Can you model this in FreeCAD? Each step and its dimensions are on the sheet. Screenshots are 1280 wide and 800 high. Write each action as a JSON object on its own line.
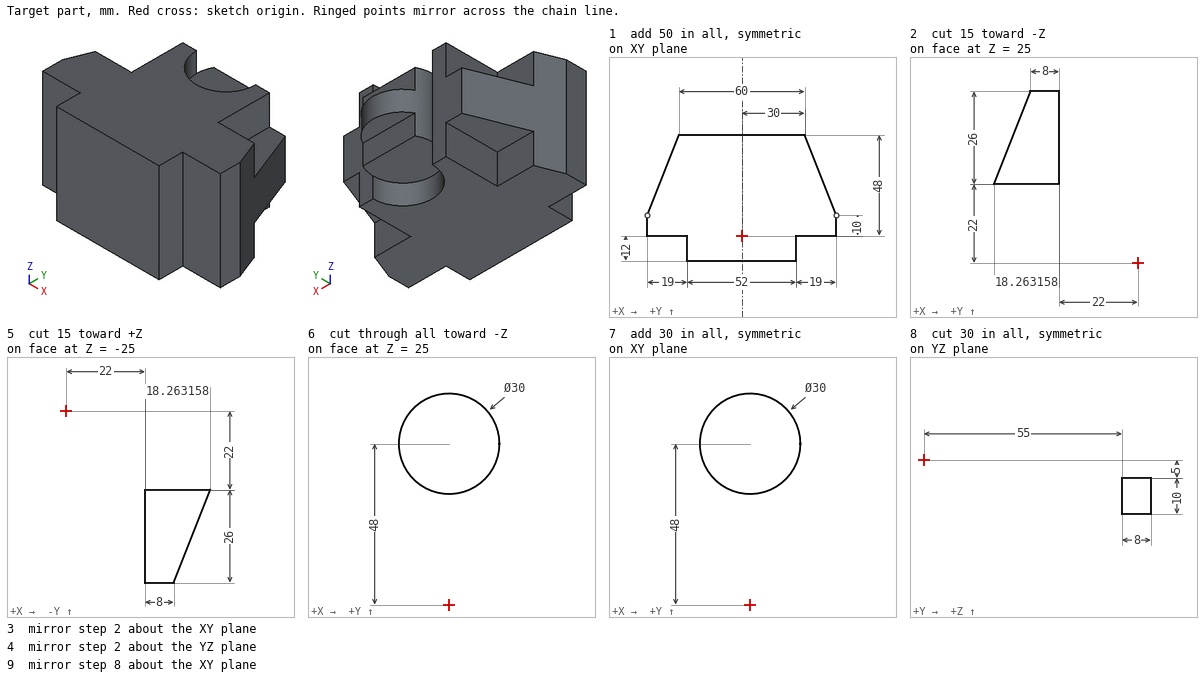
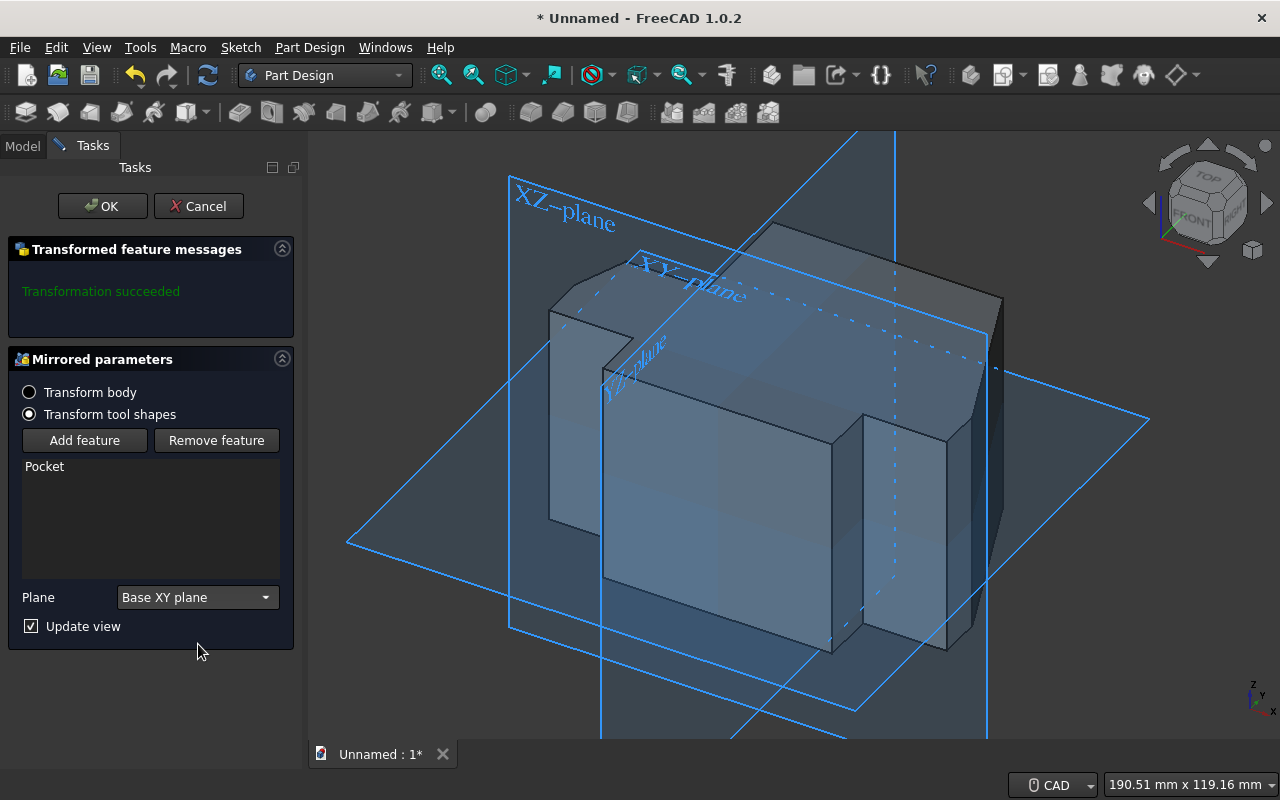
{"action": "left_click", "coordinate": [103, 206]}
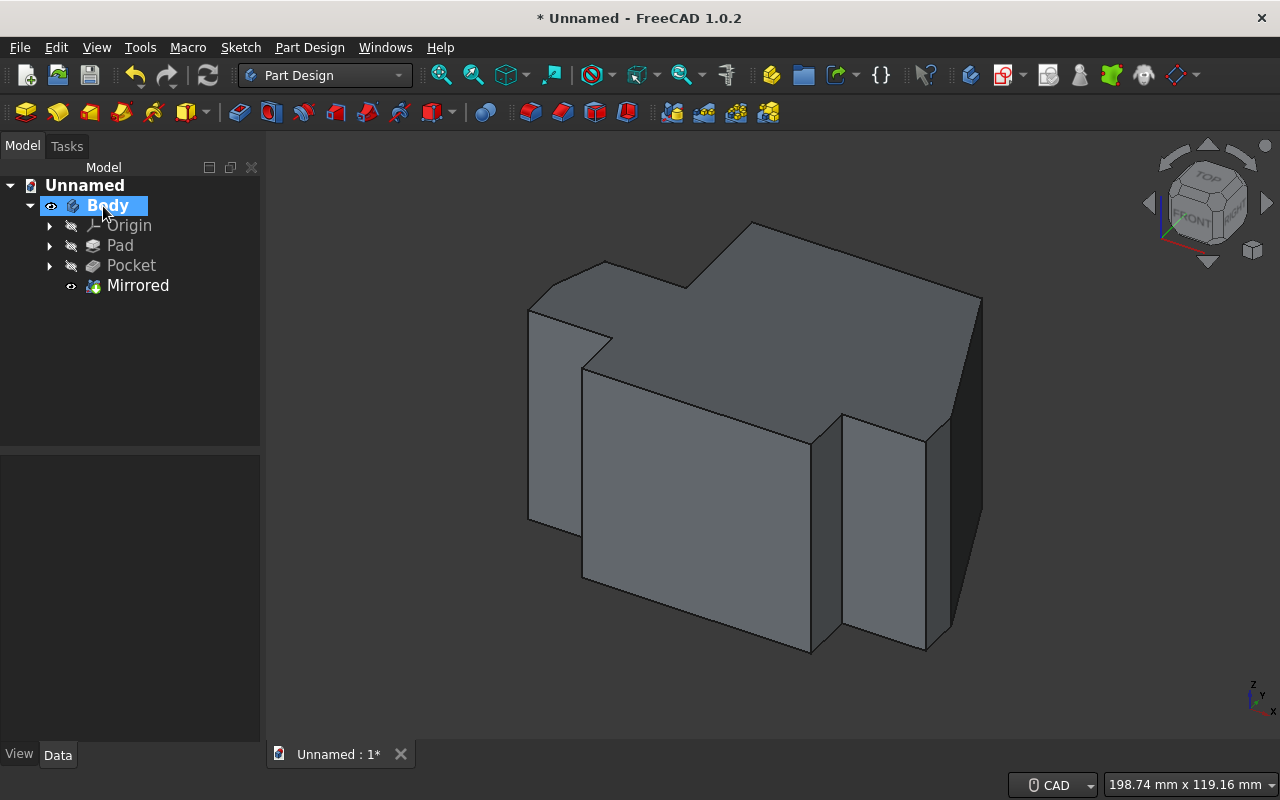
{"action": "left_click", "coordinate": [116, 266]}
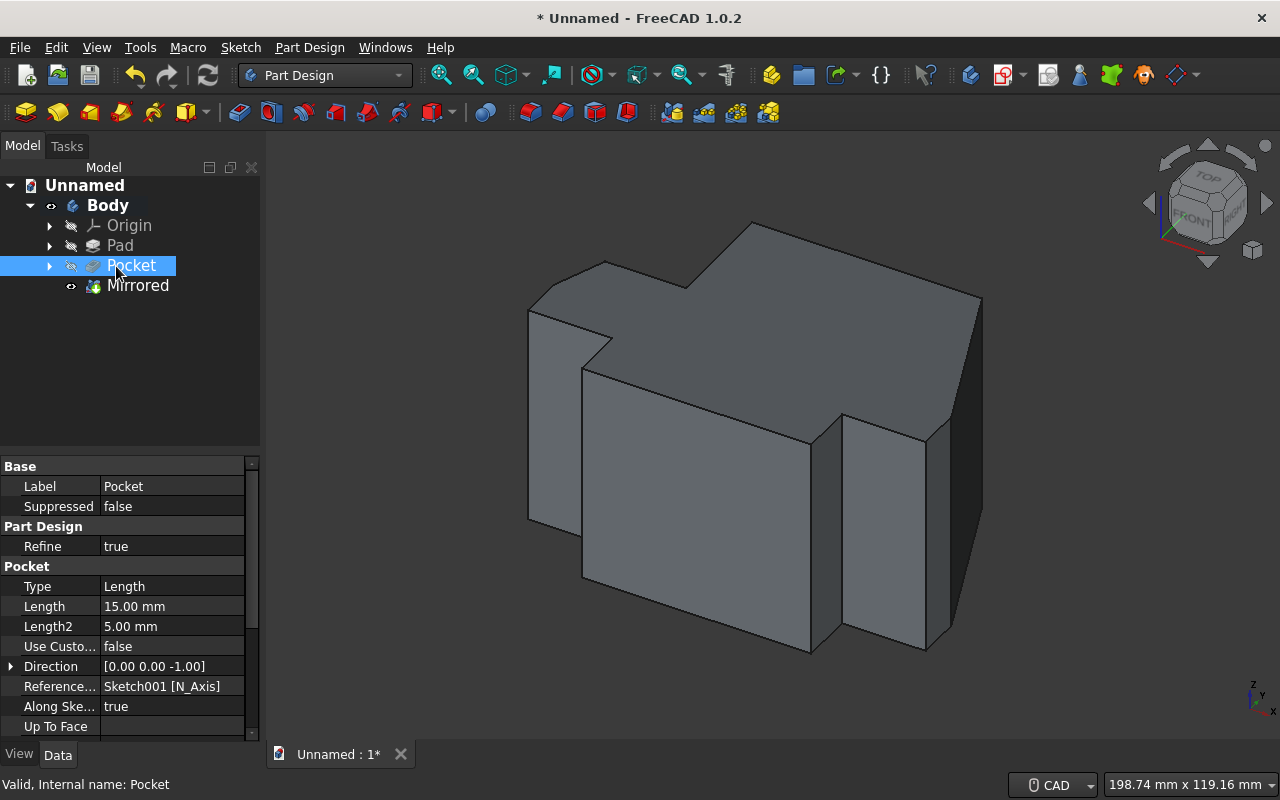
{"action": "left_click", "coordinate": [672, 112]}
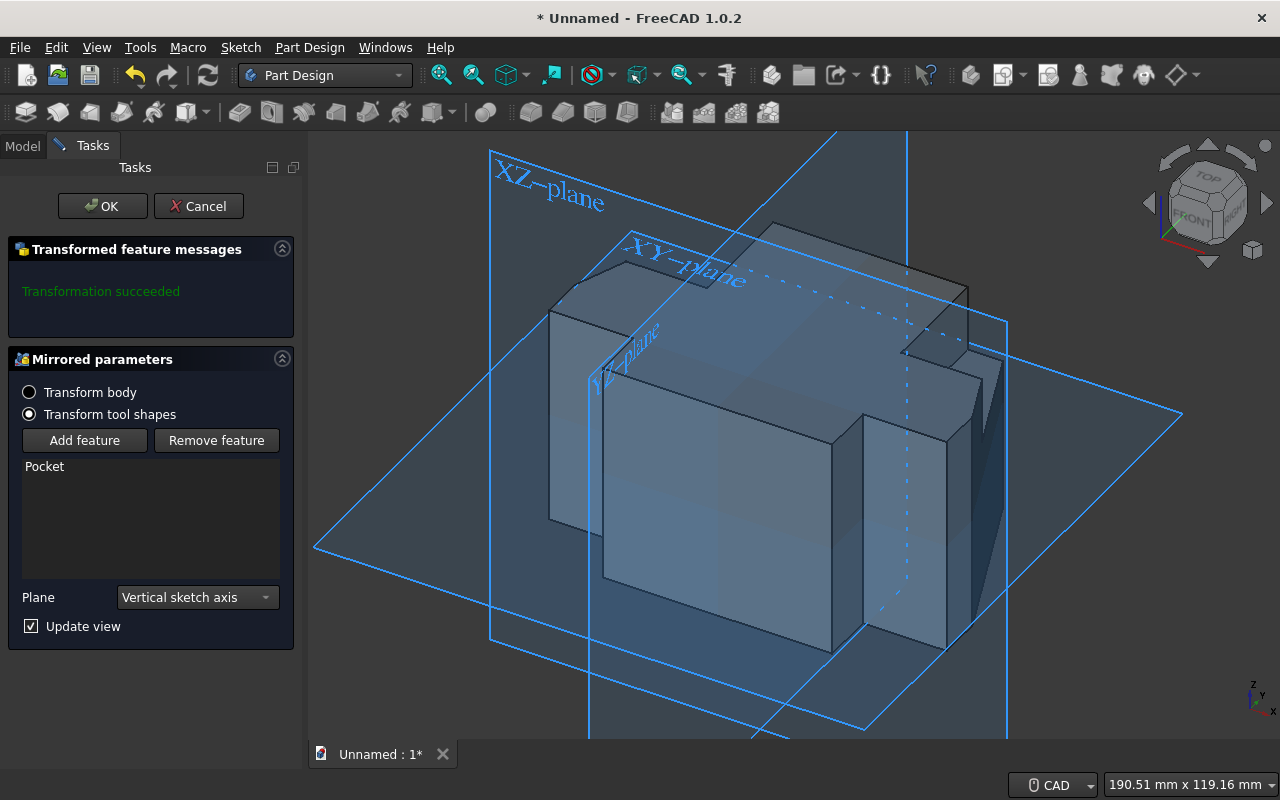
{"action": "left_click", "coordinate": [198, 598]}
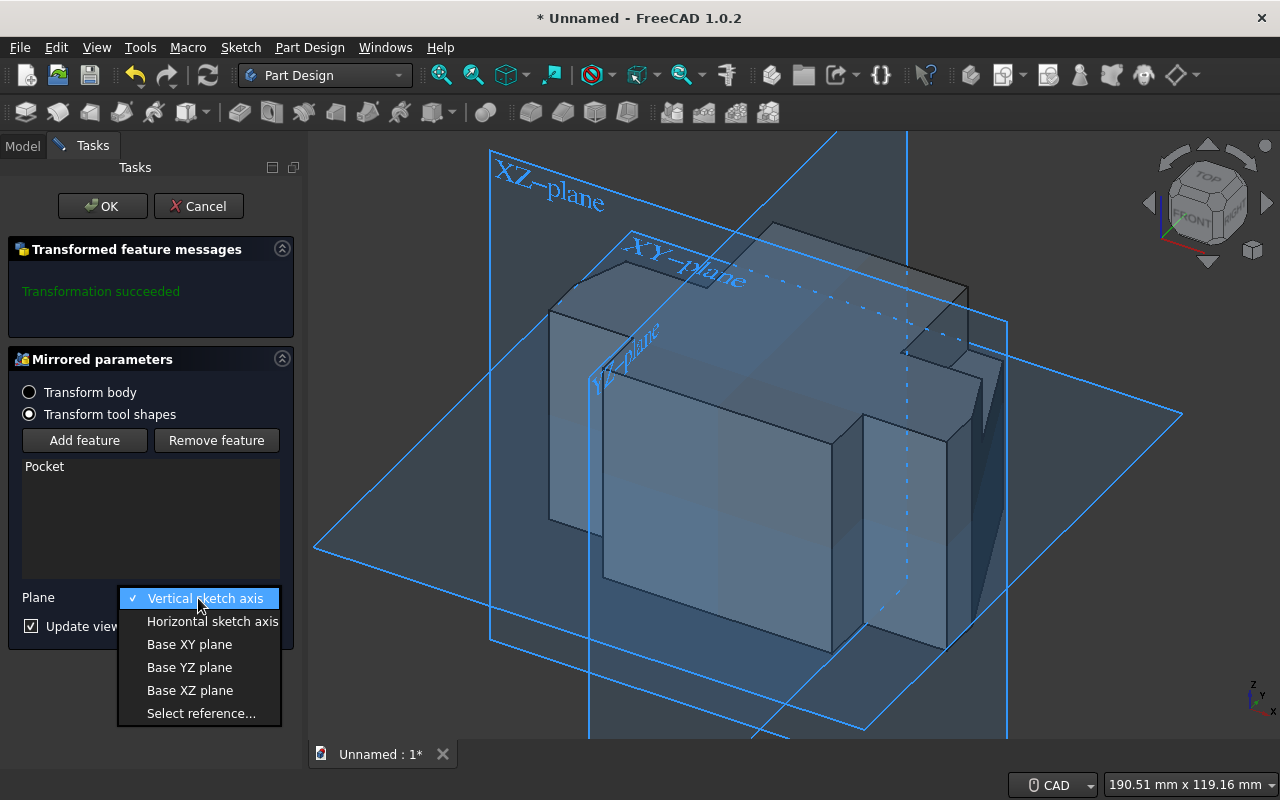
{"action": "left_click", "coordinate": [198, 668]}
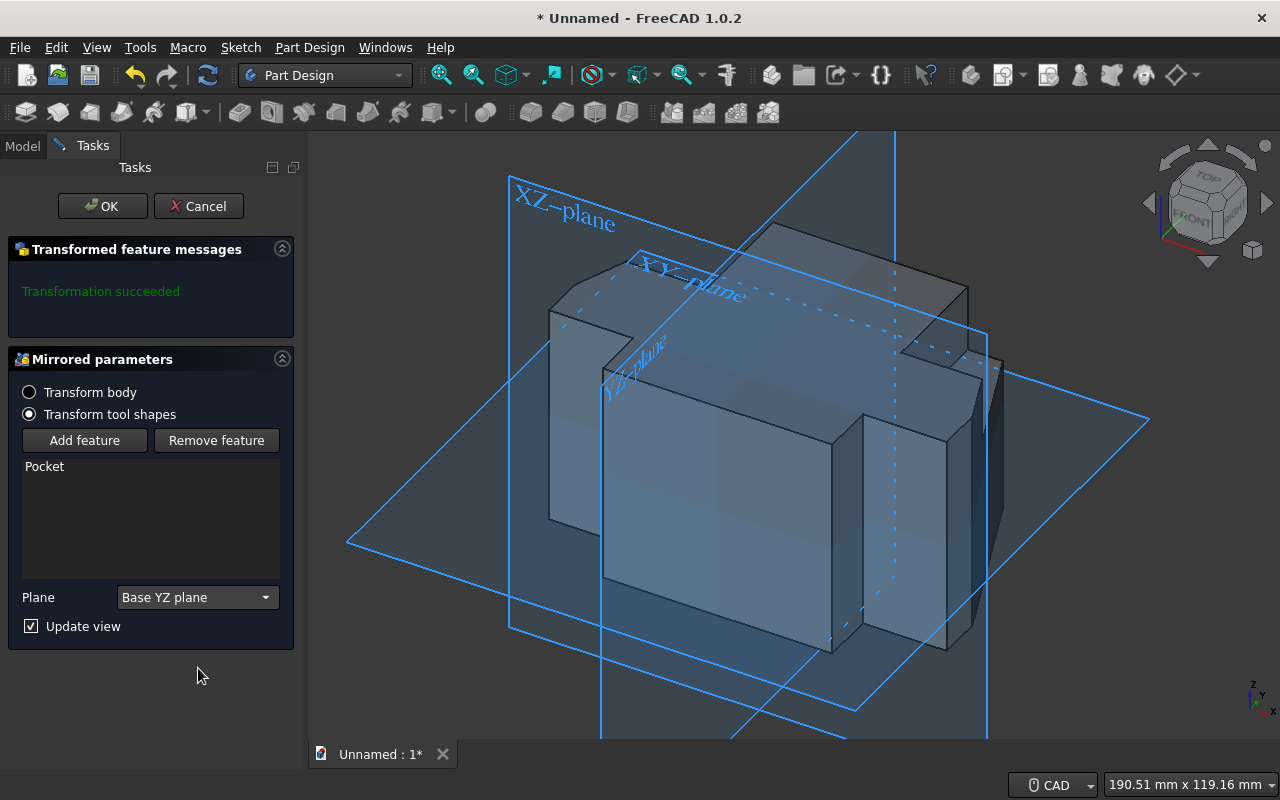
{"action": "left_click", "coordinate": [103, 206]}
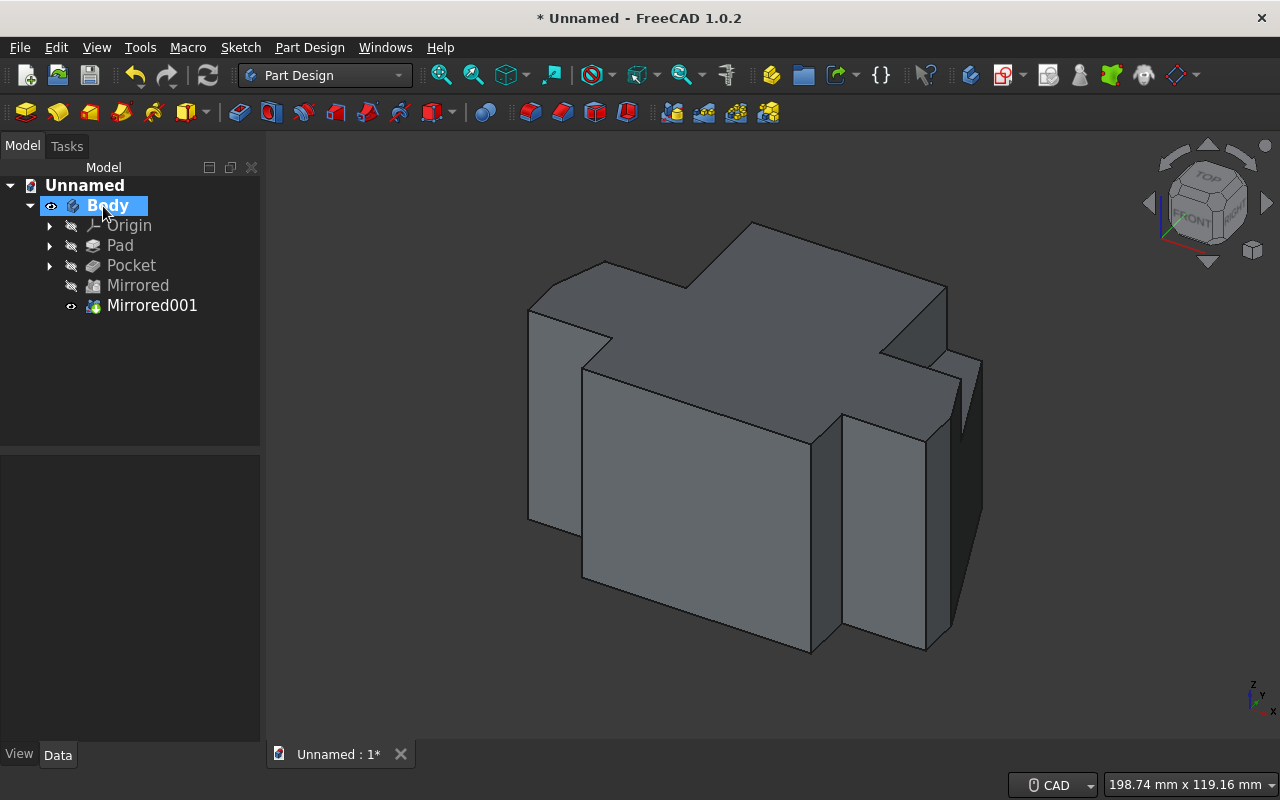
{"action": "key", "text": "5"}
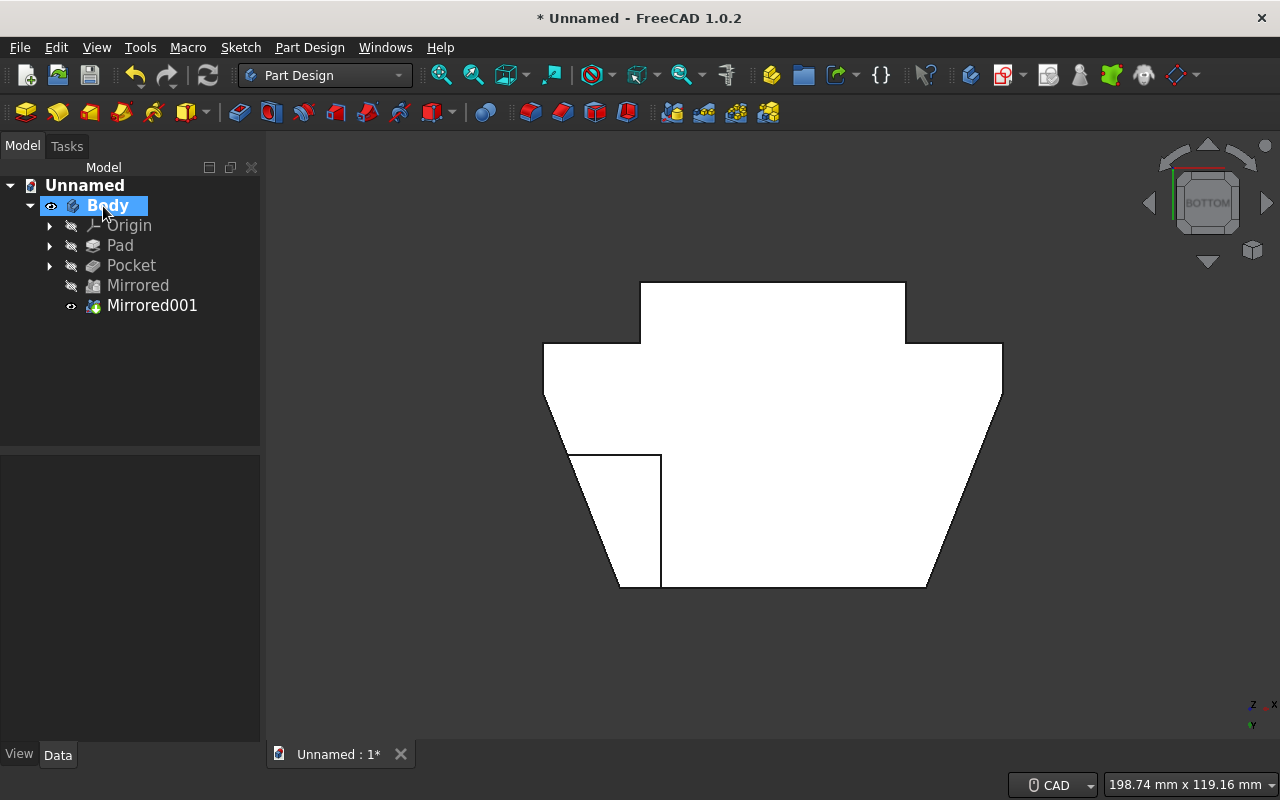
{"action": "left_click", "coordinate": [773, 434]}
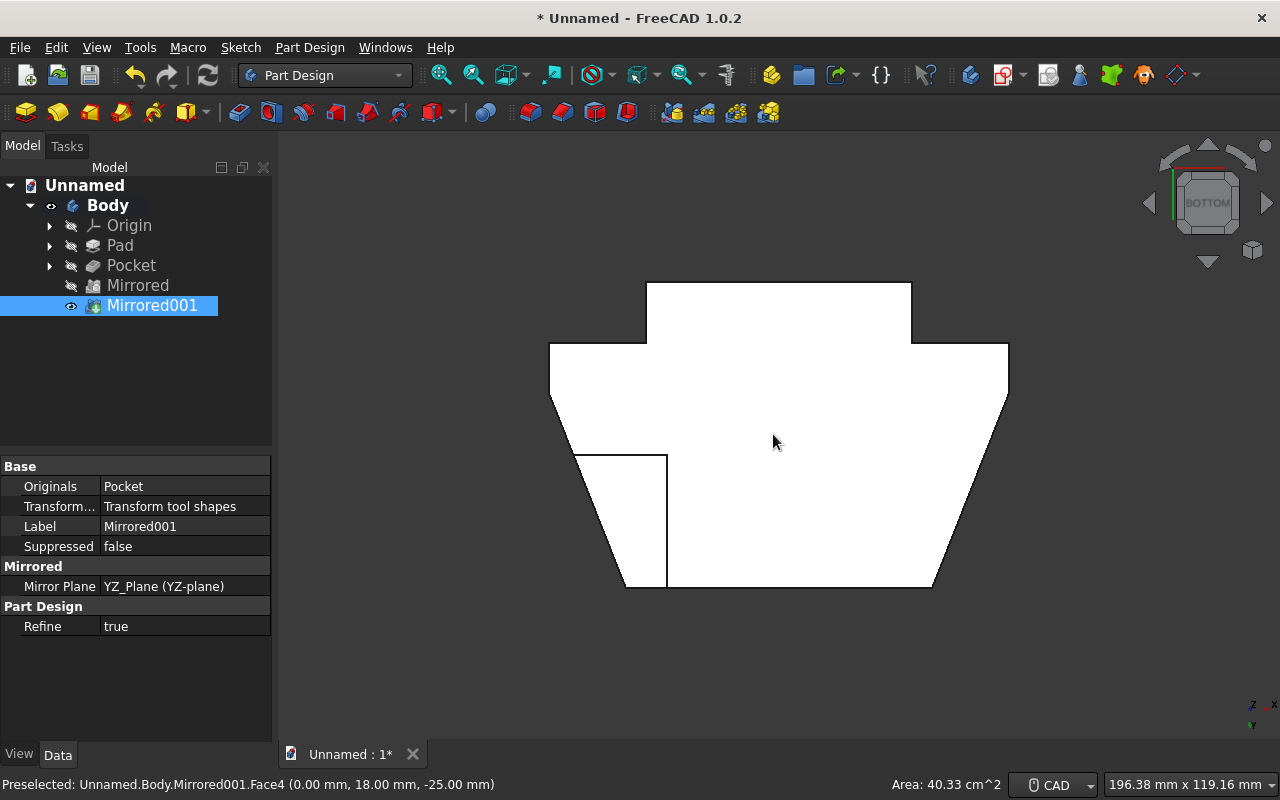
{"action": "left_click", "coordinate": [1004, 76]}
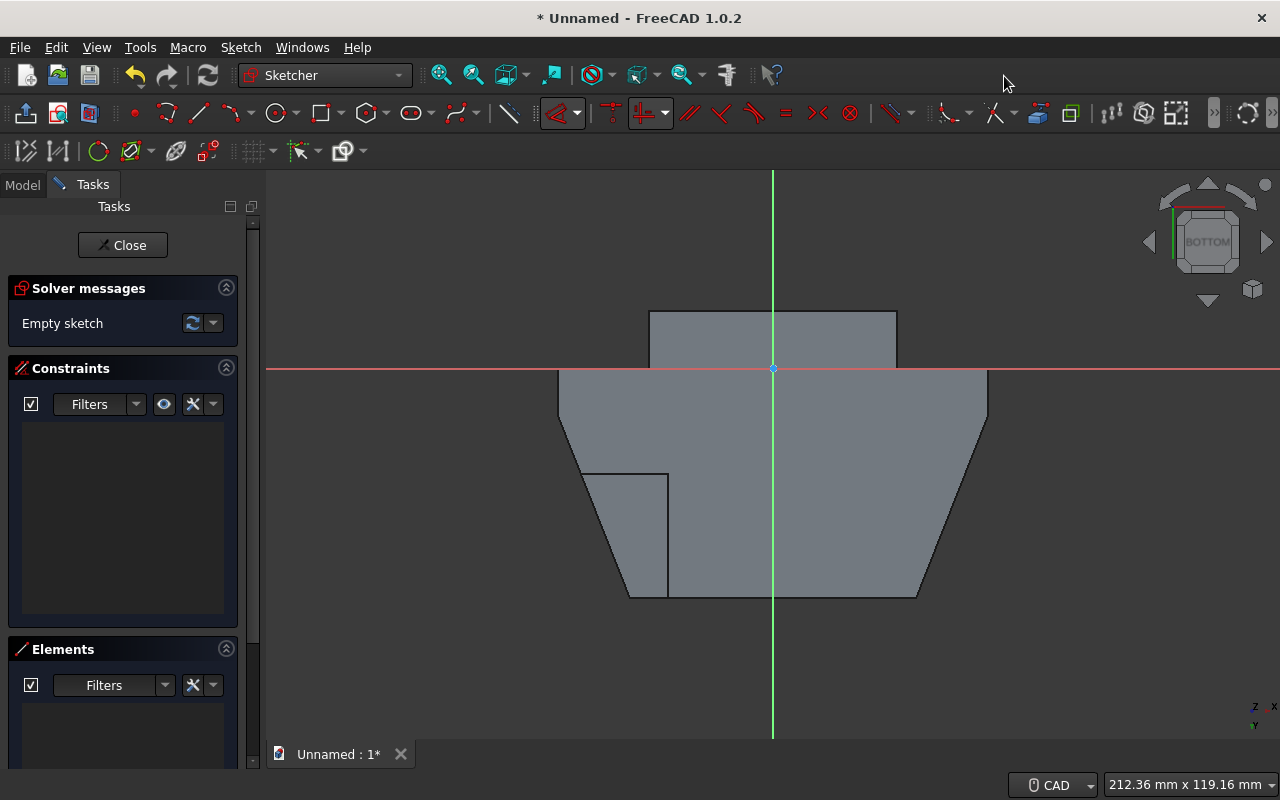
{"action": "scroll", "coordinate": [1115, 541], "scroll_direction": "up", "scroll_amount": 2}